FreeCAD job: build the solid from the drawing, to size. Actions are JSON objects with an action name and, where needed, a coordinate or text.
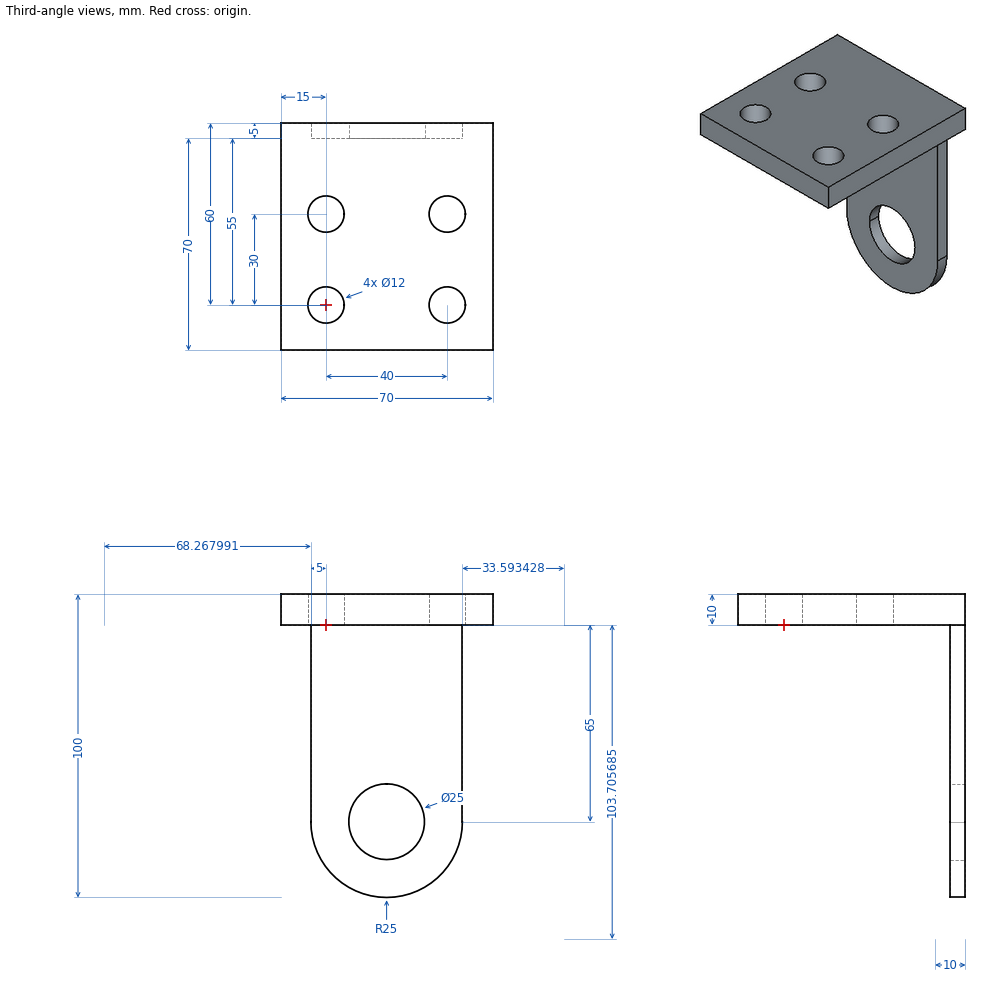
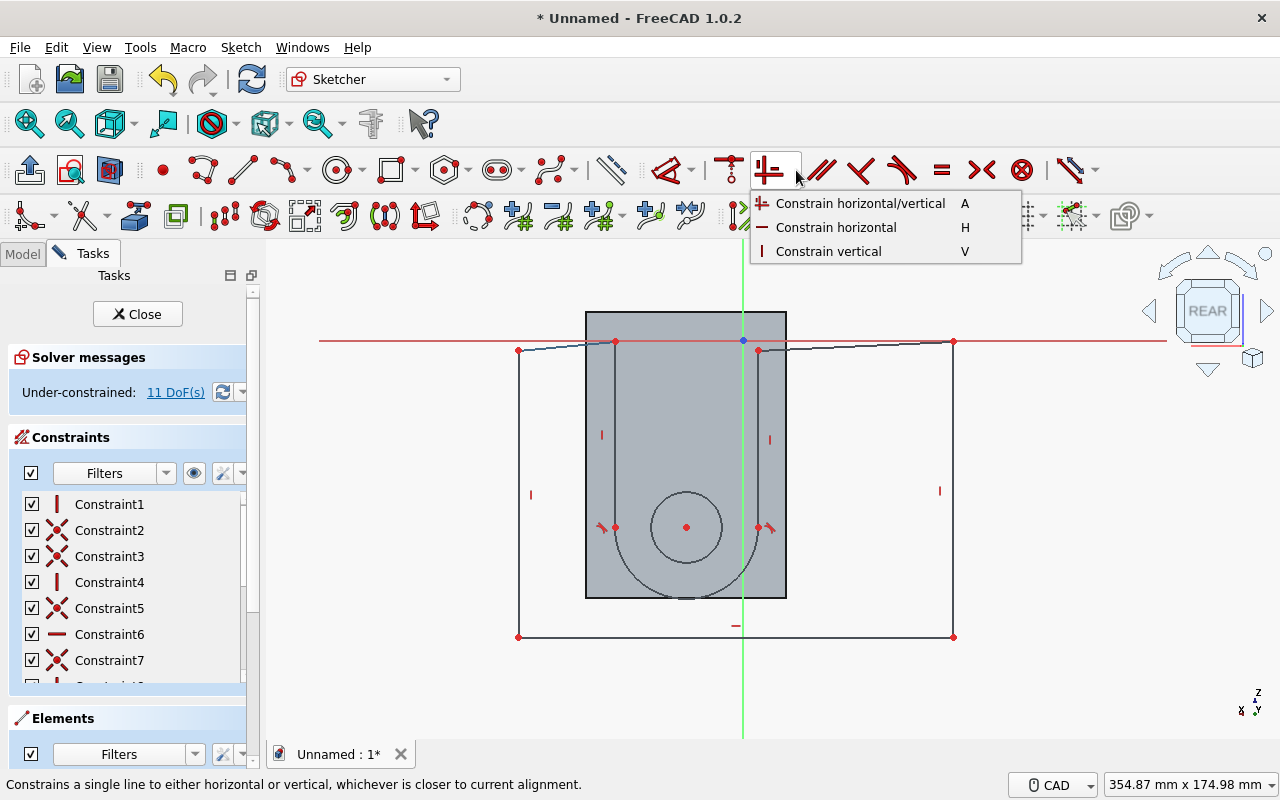
{"action": "left_click", "coordinate": [886, 227]}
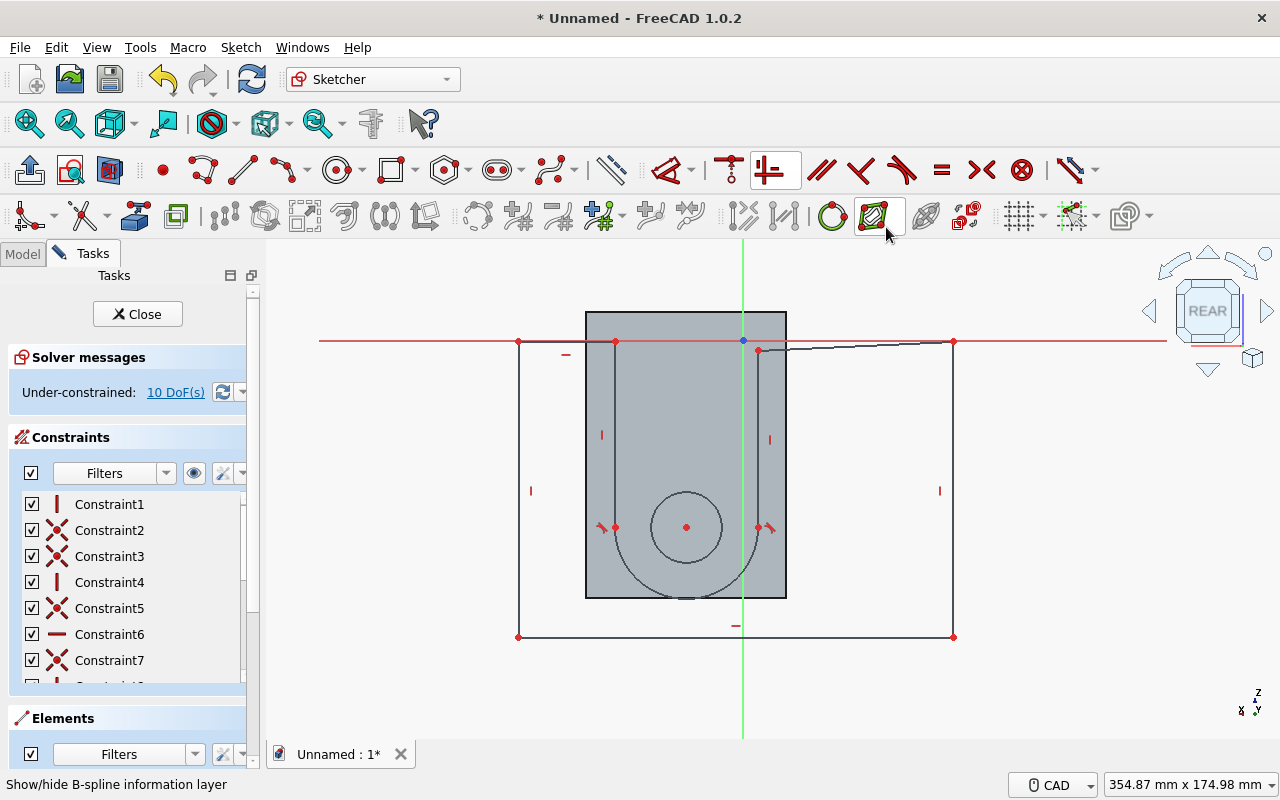
{"action": "left_click", "coordinate": [895, 345]}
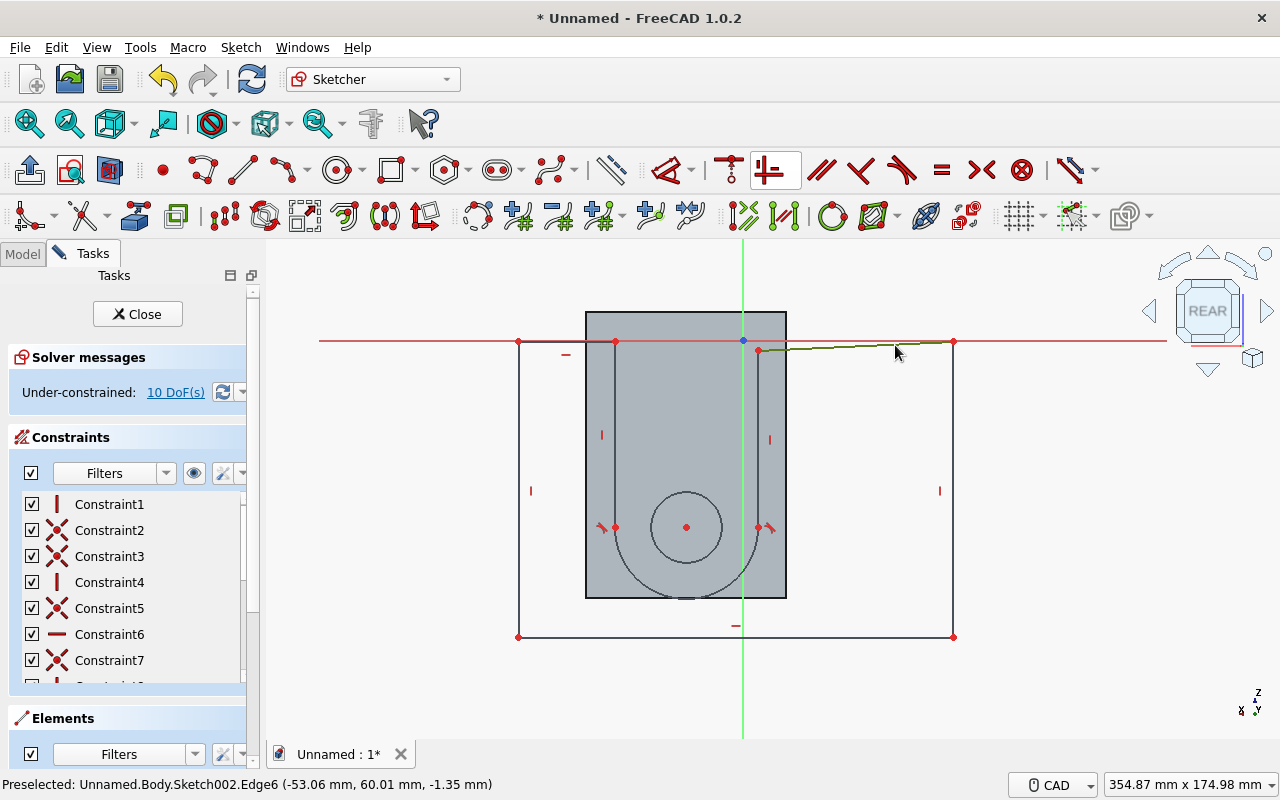
{"action": "left_click", "coordinate": [796, 170]}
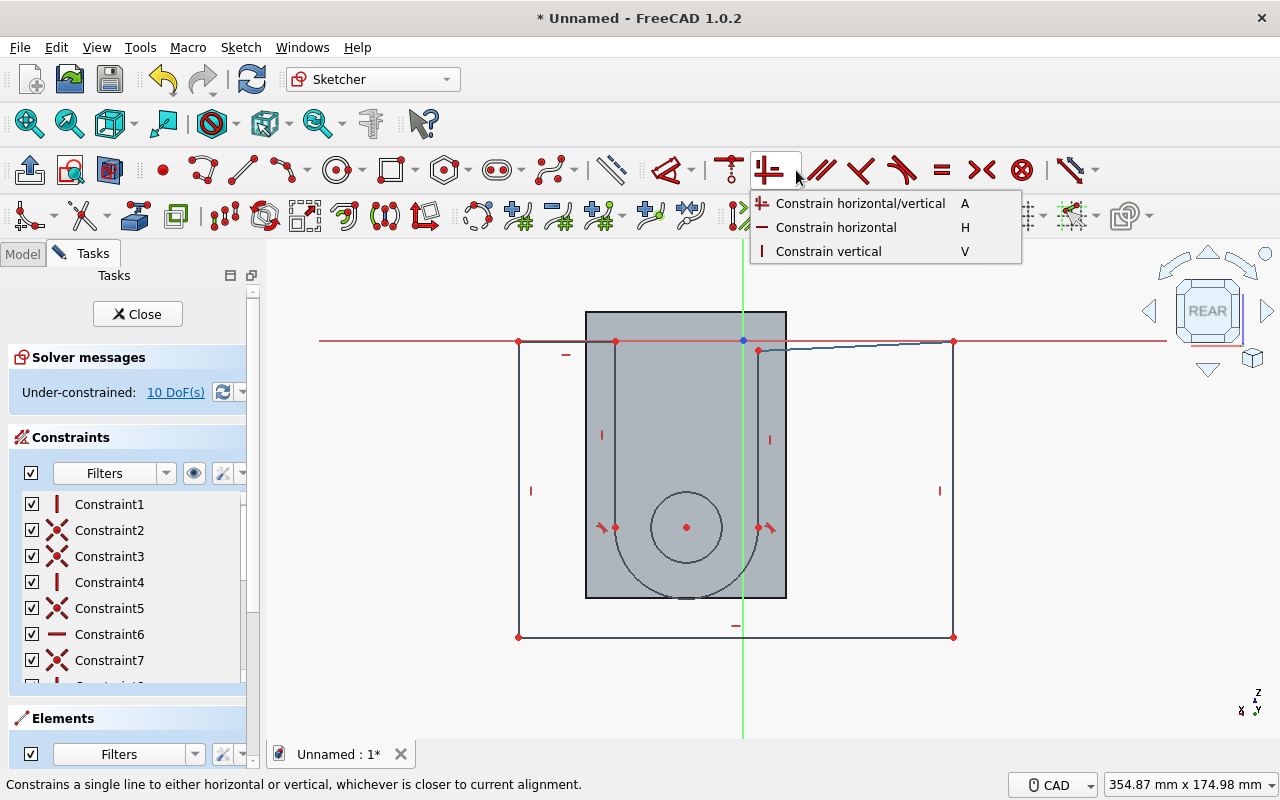
{"action": "left_click", "coordinate": [886, 227]}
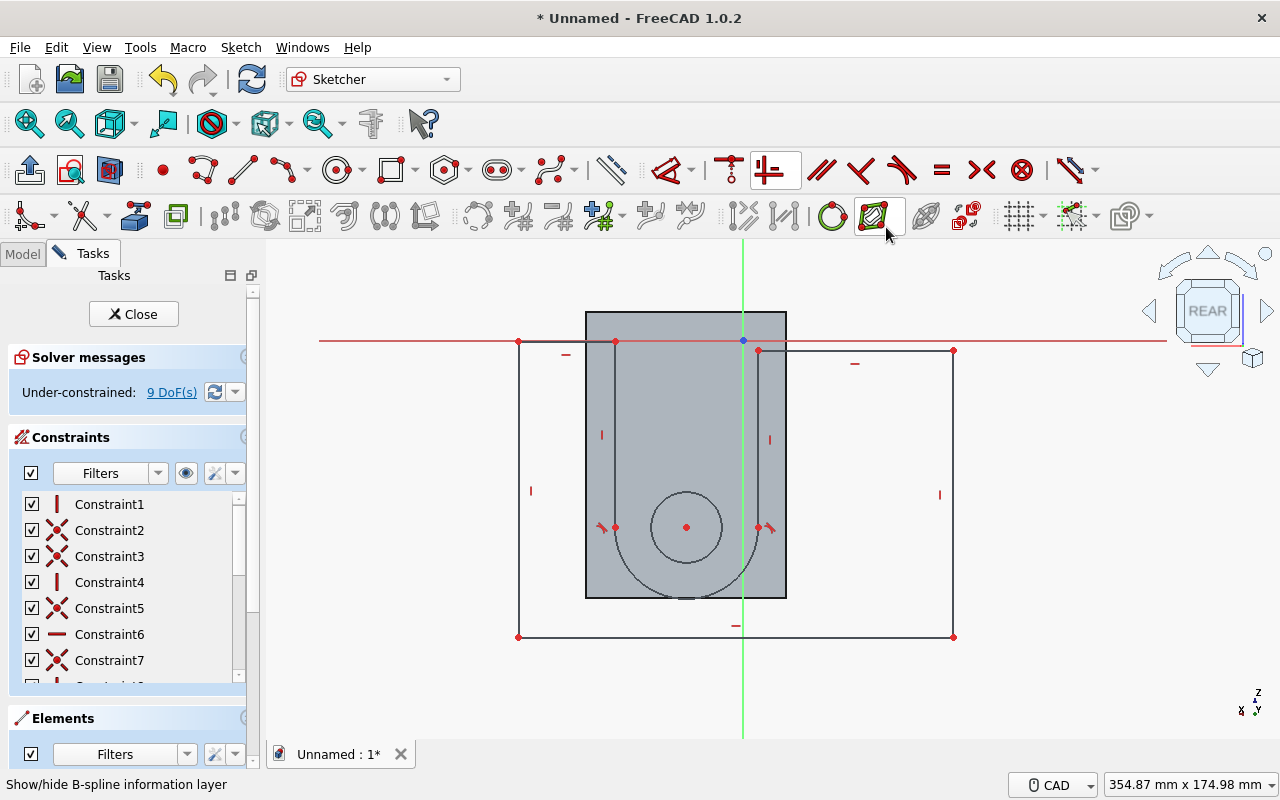
{"action": "left_click", "coordinate": [666, 170]}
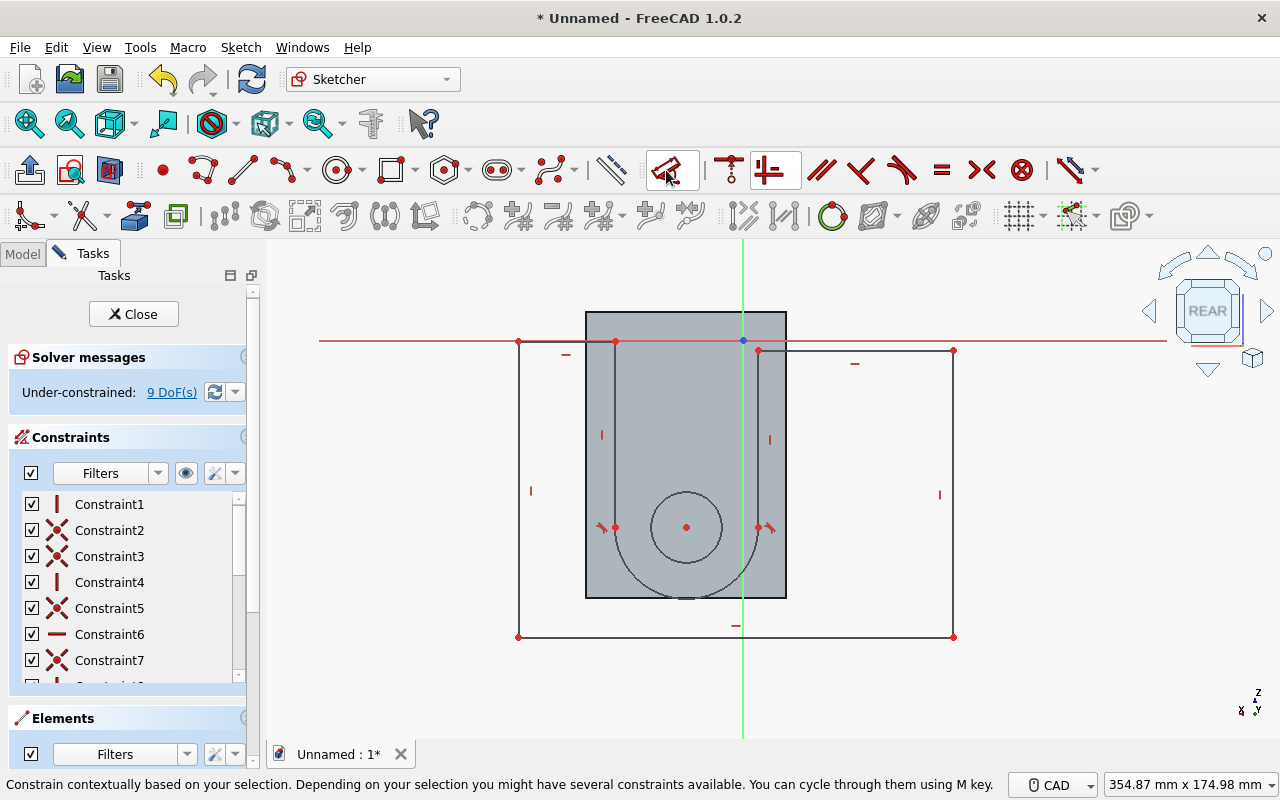
{"action": "left_click", "coordinate": [644, 585]}
{"action": "left_click", "coordinate": [625, 611]}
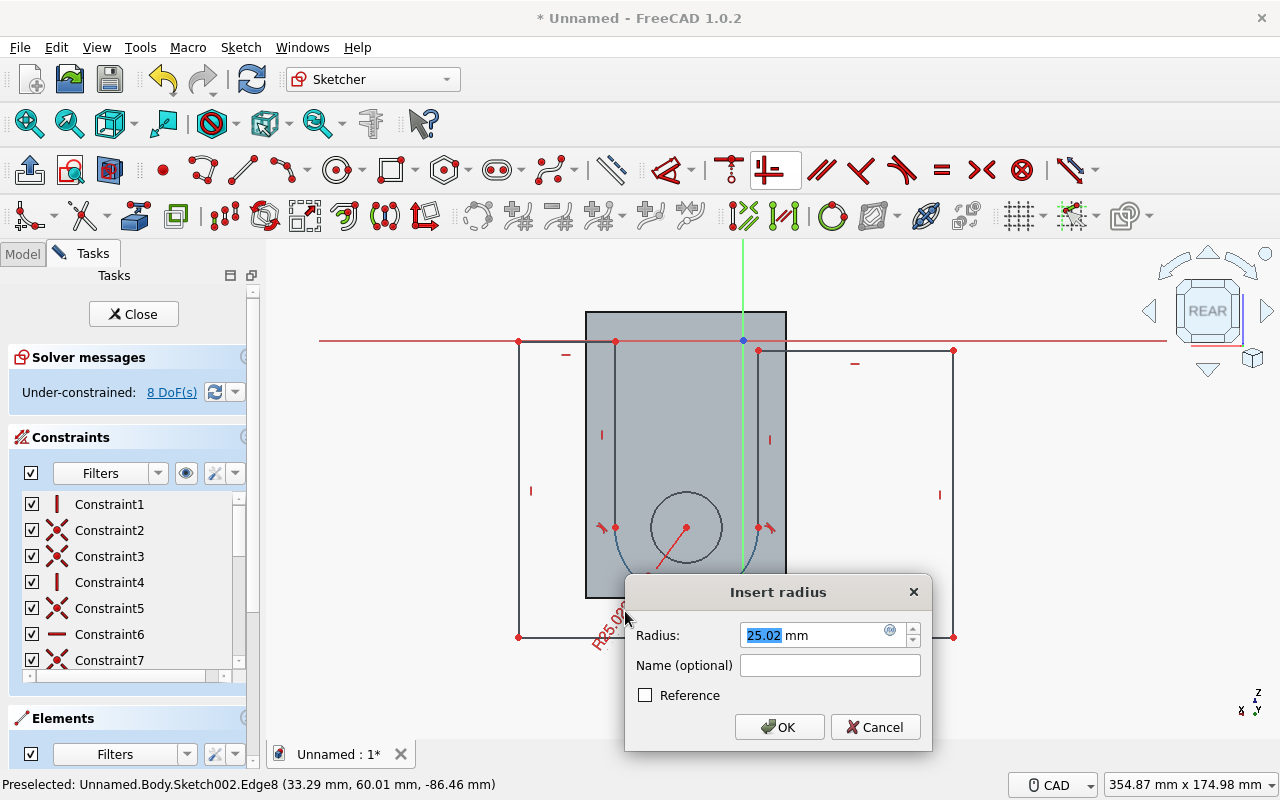
{"action": "type", "text": "25"}
{"action": "key", "text": "Return"}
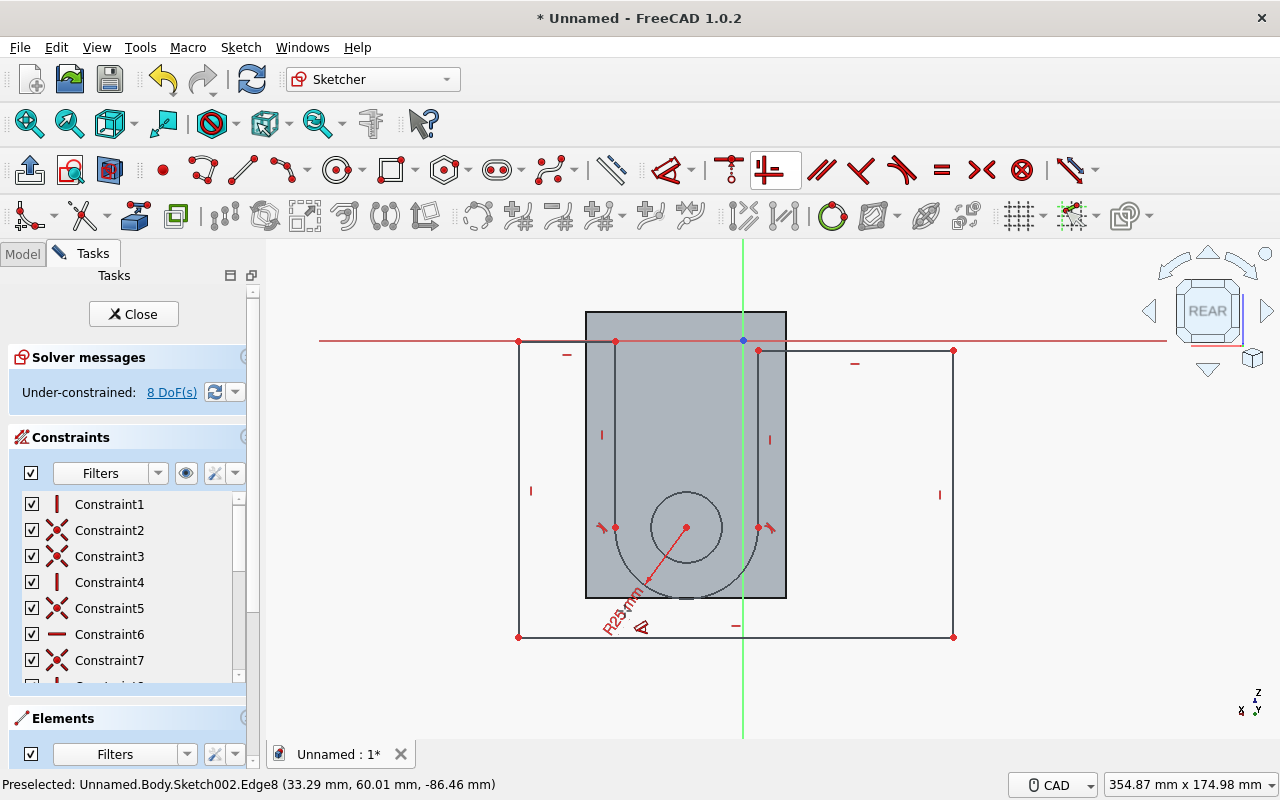
{"action": "left_click", "coordinate": [711, 502]}
{"action": "left_click", "coordinate": [704, 463]}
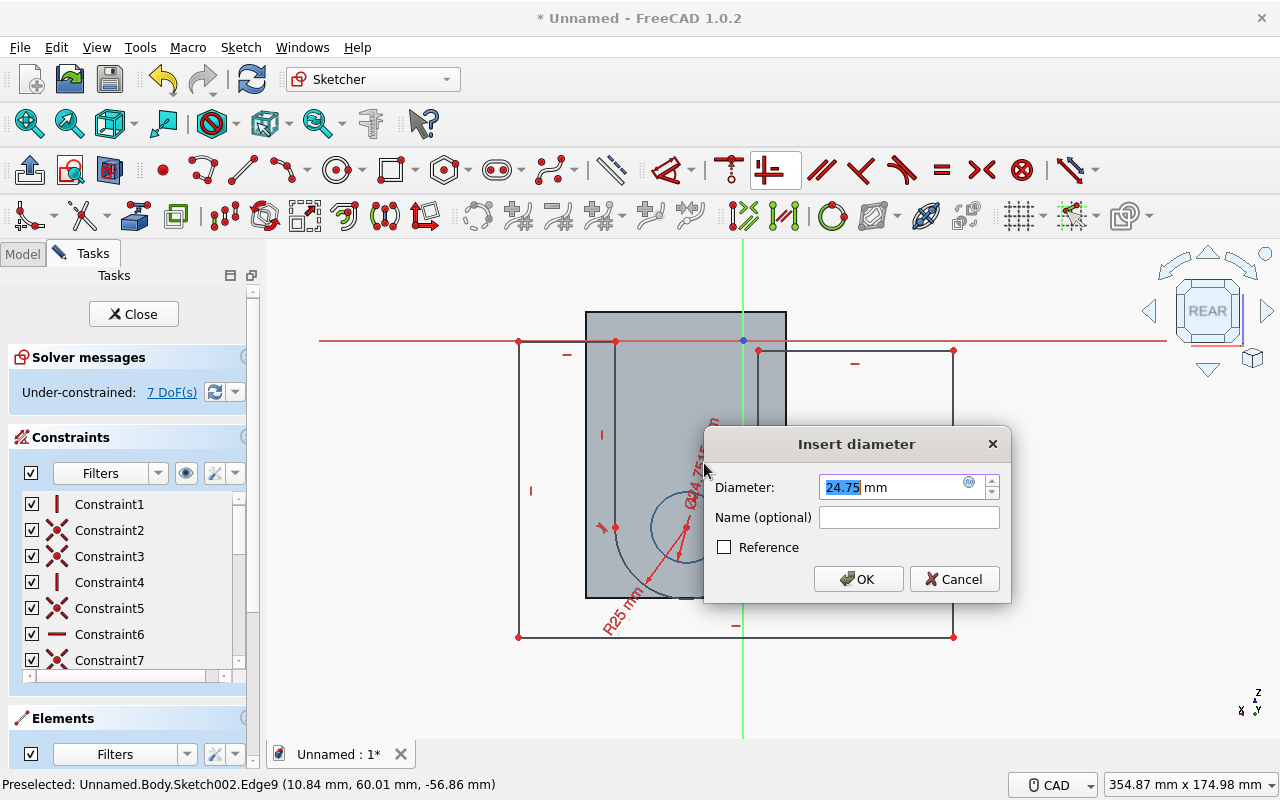
{"action": "type", "text": "25"}
{"action": "key", "text": "Return"}
{"action": "key", "text": "Escape"}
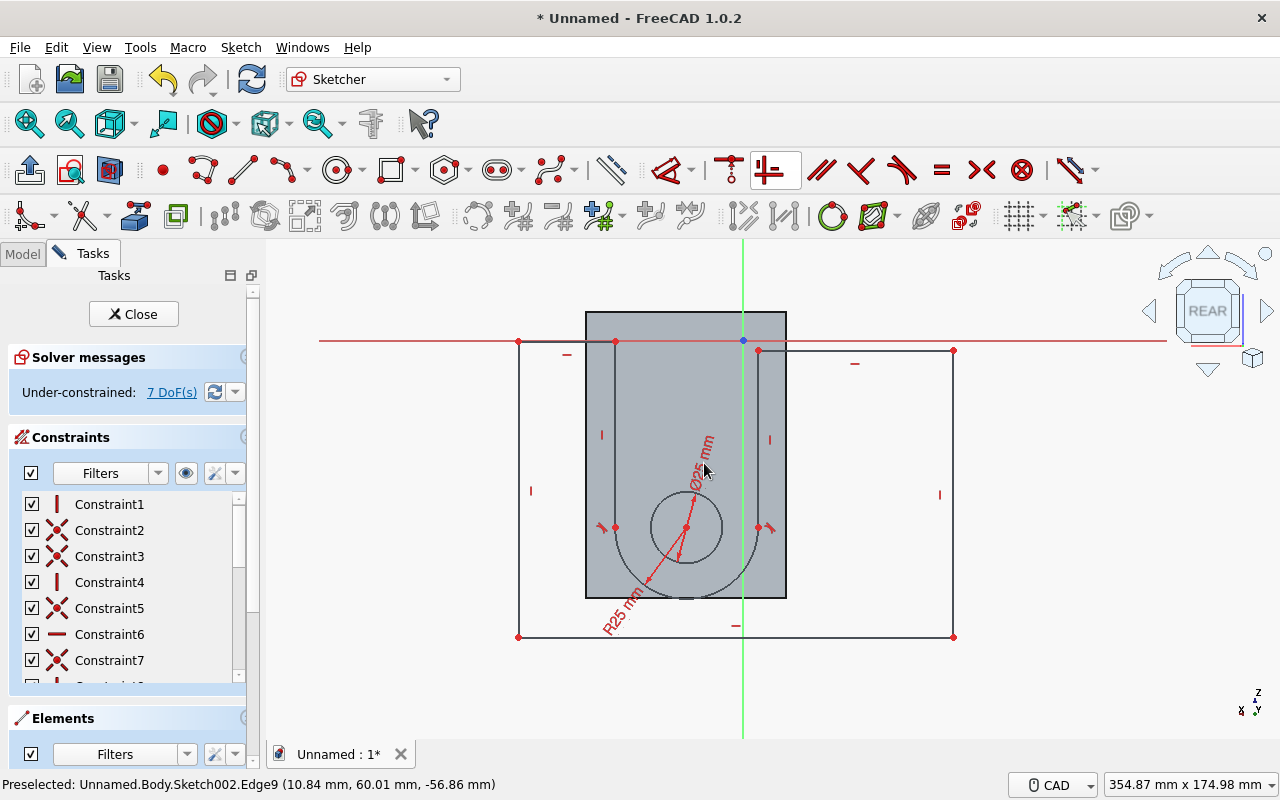
{"action": "left_click", "coordinate": [615, 342]}